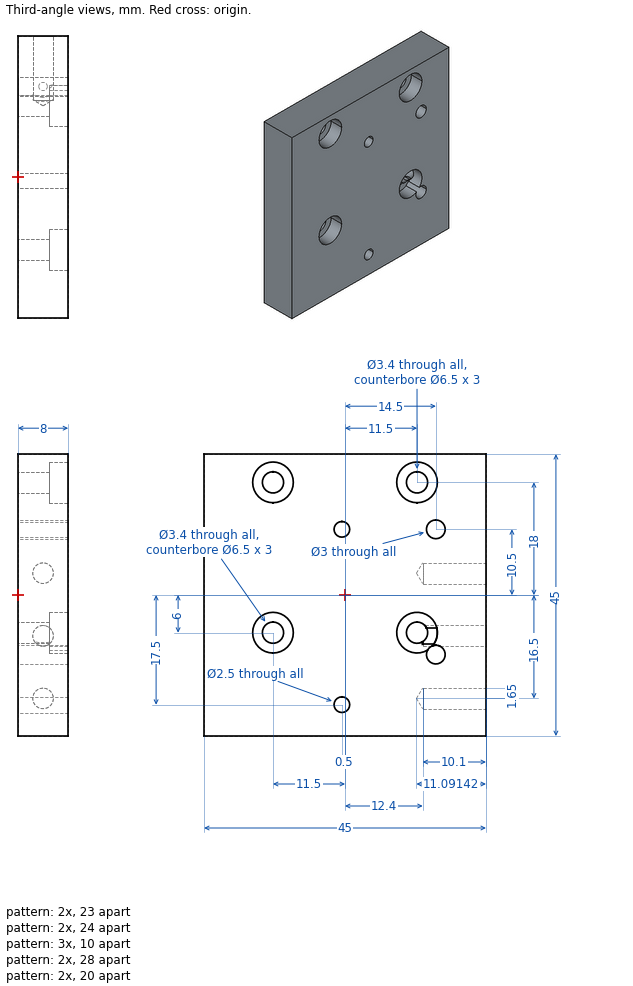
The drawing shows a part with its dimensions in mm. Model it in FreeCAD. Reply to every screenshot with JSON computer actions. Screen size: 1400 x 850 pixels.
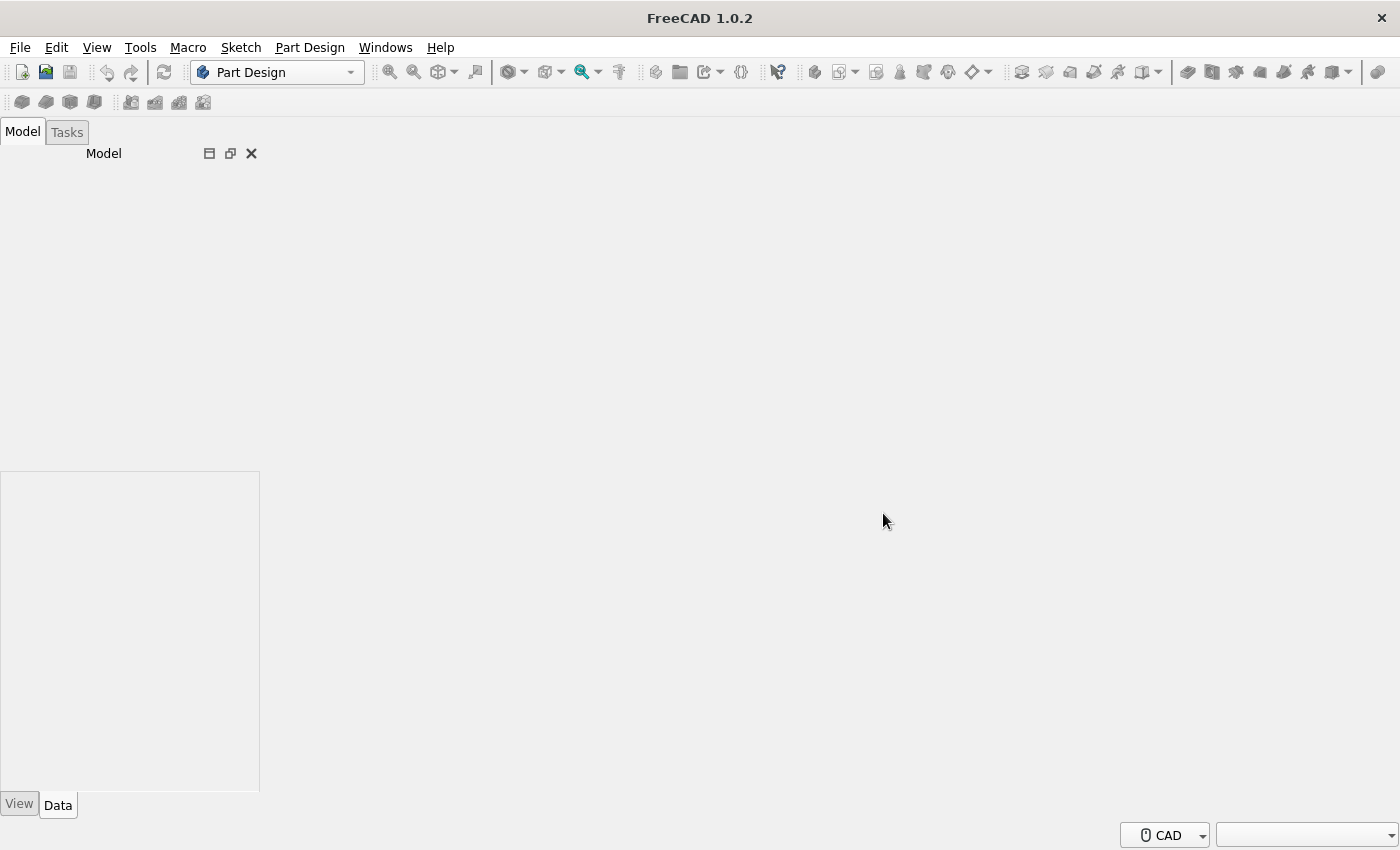
{"action": "key", "text": "ctrl+n"}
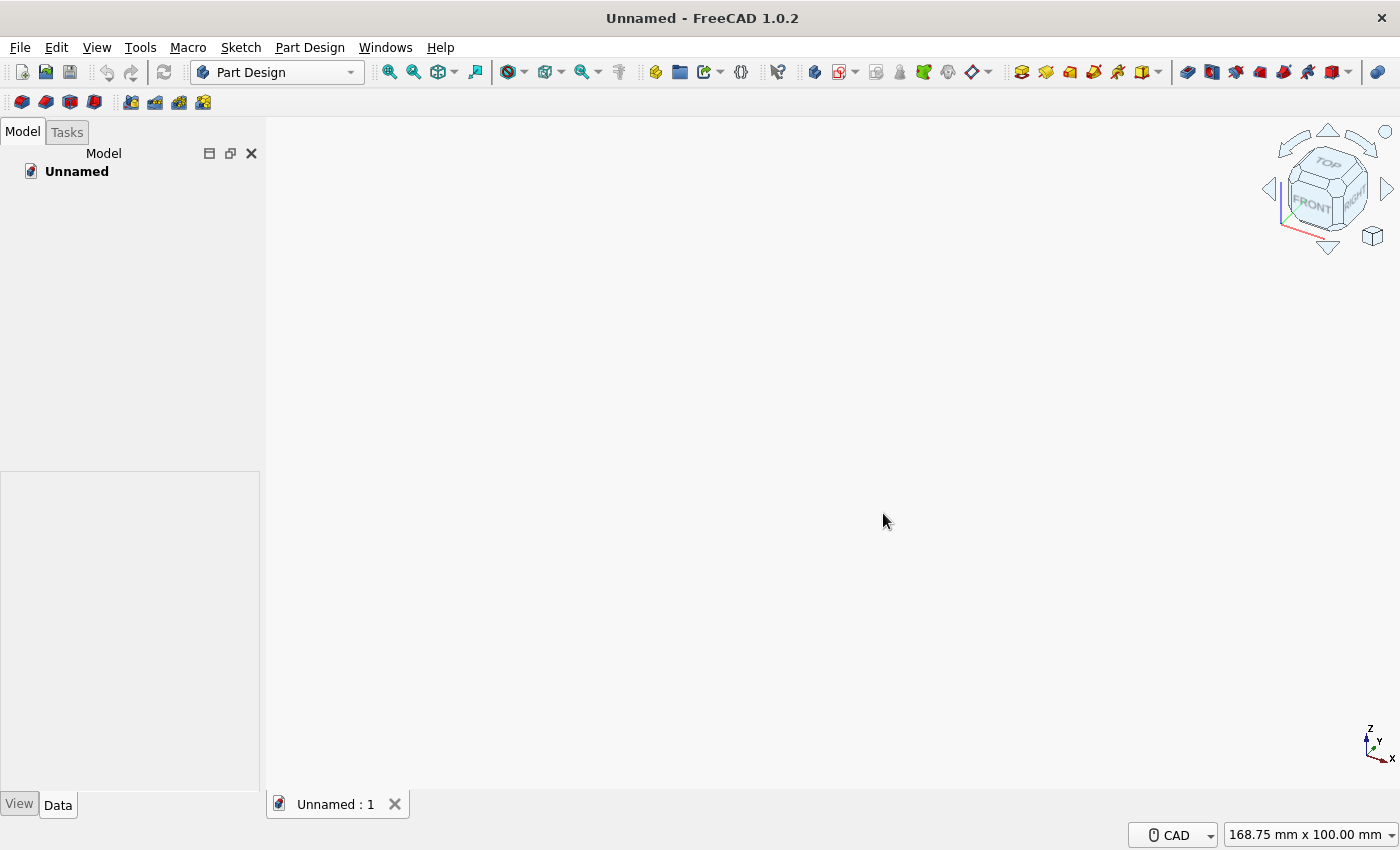
{"action": "left_click", "coordinate": [840, 72]}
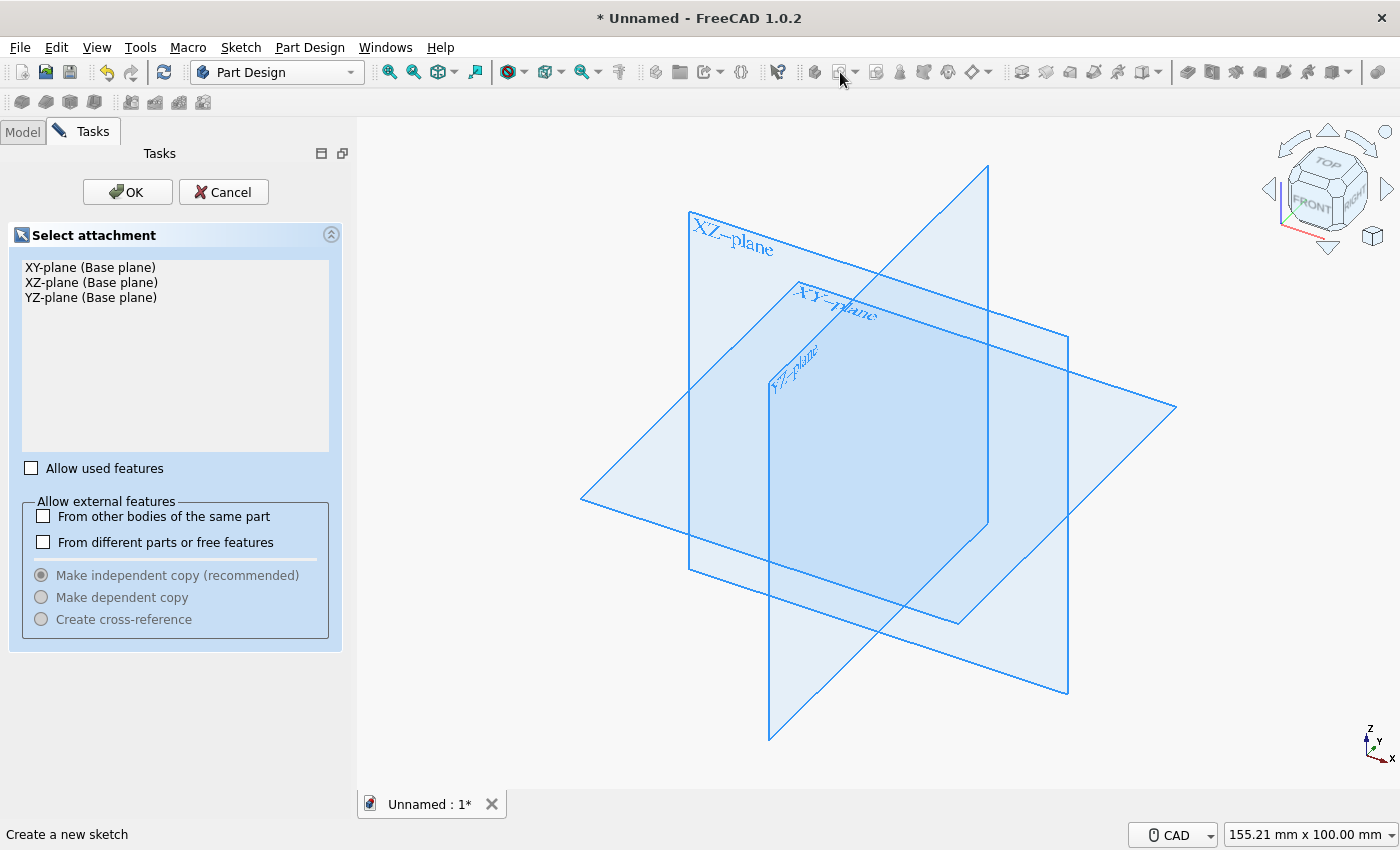
{"action": "left_click", "coordinate": [82, 298]}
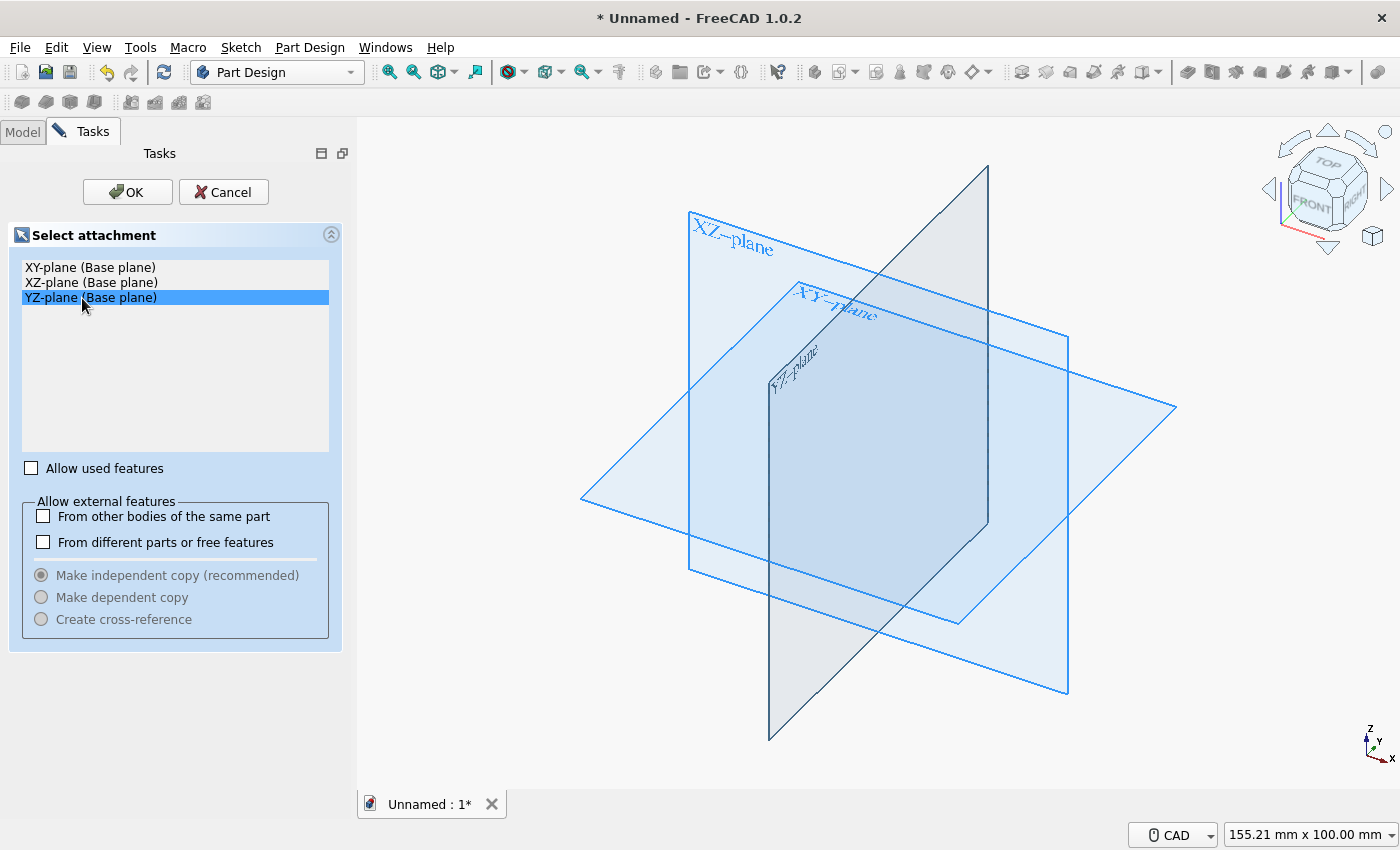
{"action": "left_click", "coordinate": [128, 192]}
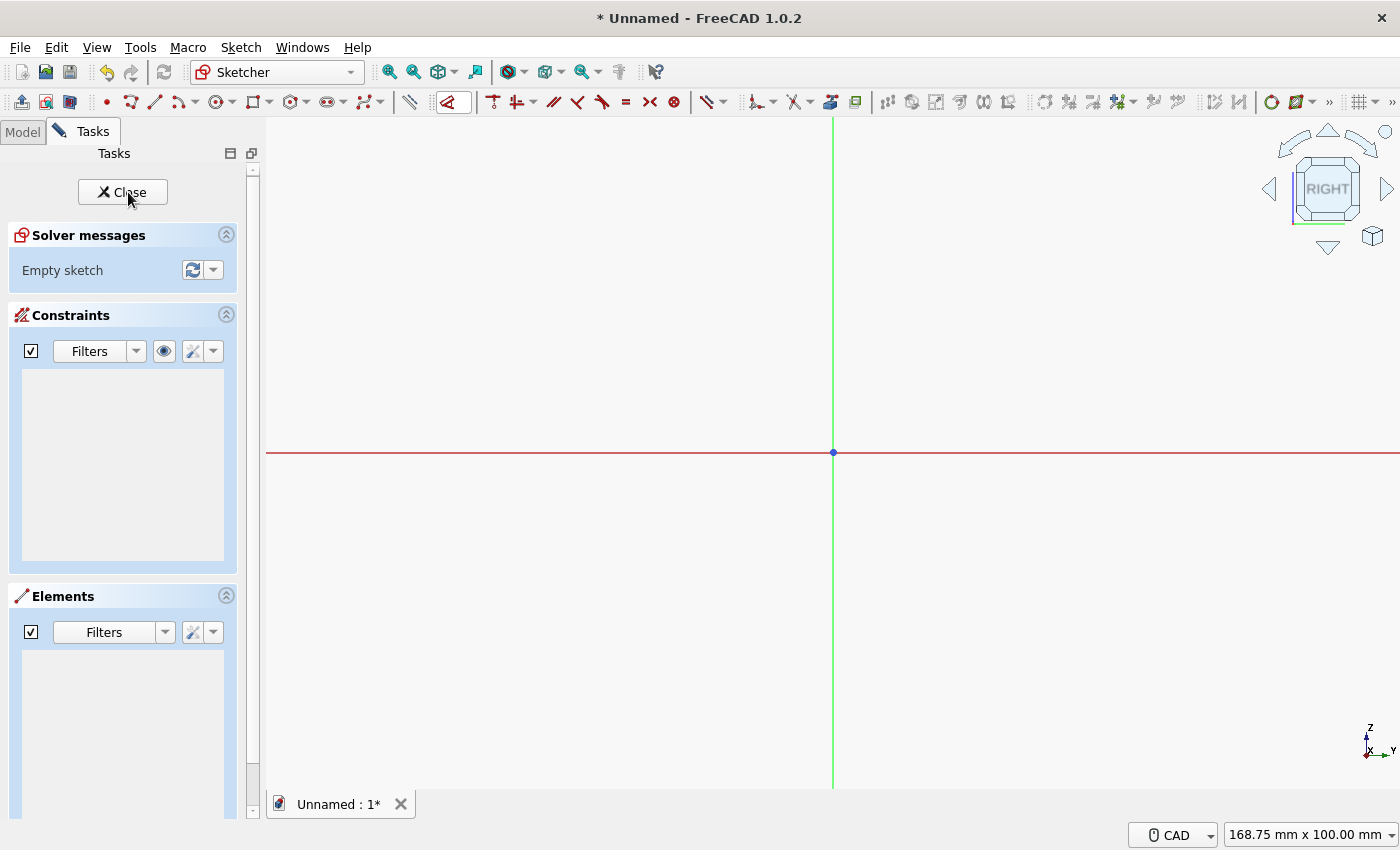
{"action": "scroll", "coordinate": [972, 453], "scroll_direction": "up", "scroll_amount": 2}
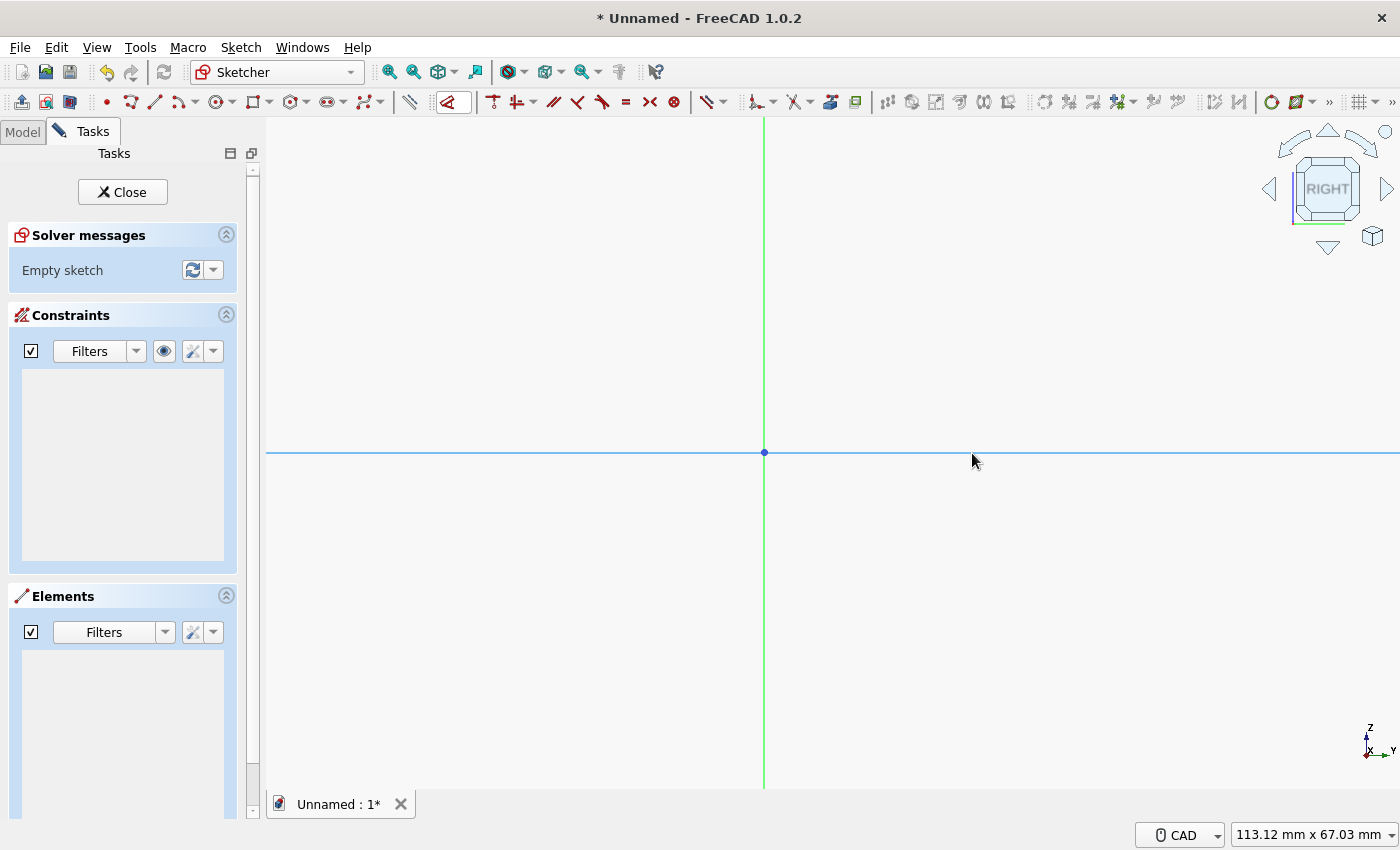
{"action": "key", "text": "g v"}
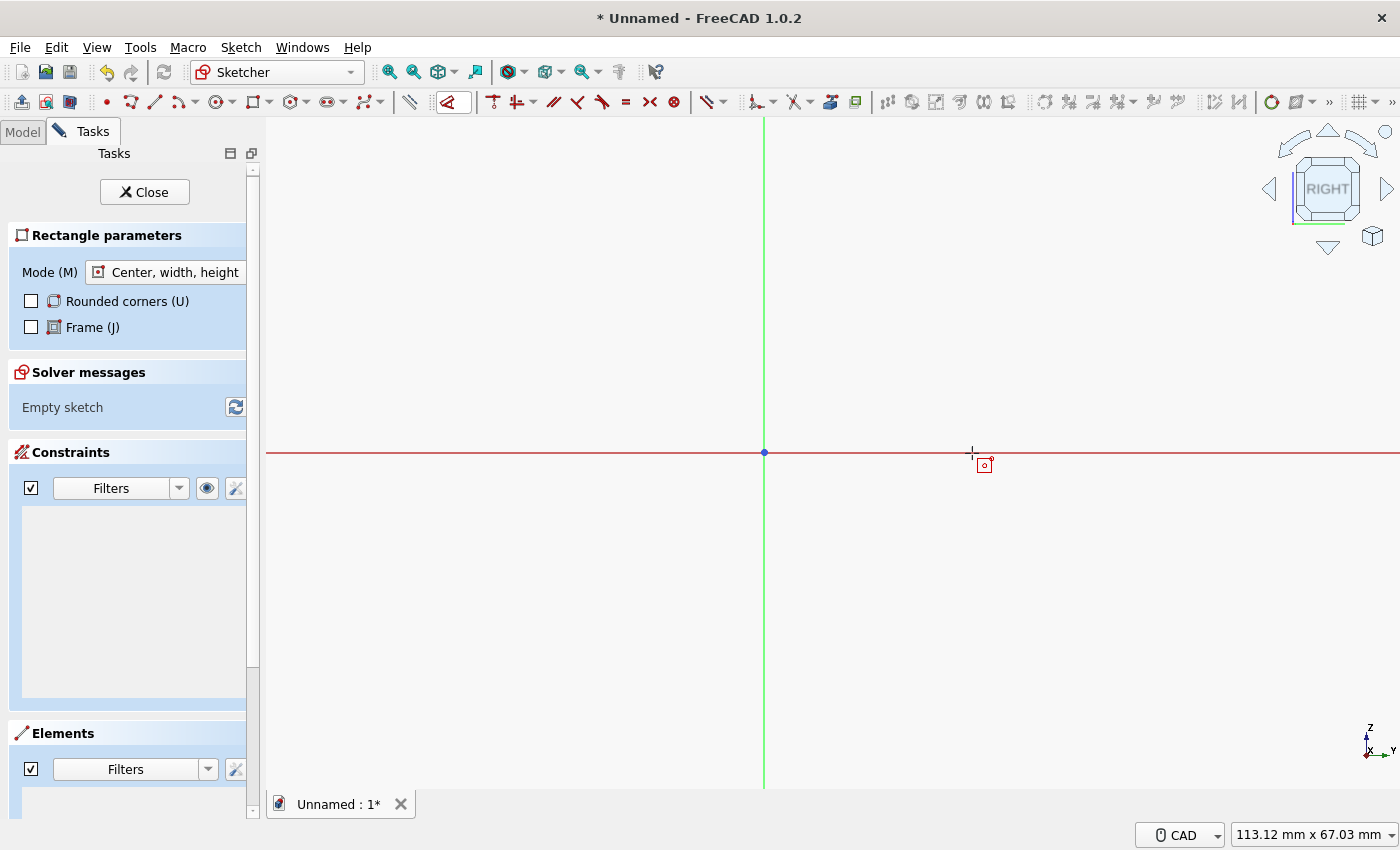
{"action": "left_click", "coordinate": [764, 453]}
{"action": "left_click", "coordinate": [990, 227]}
{"action": "key", "text": "Escape"}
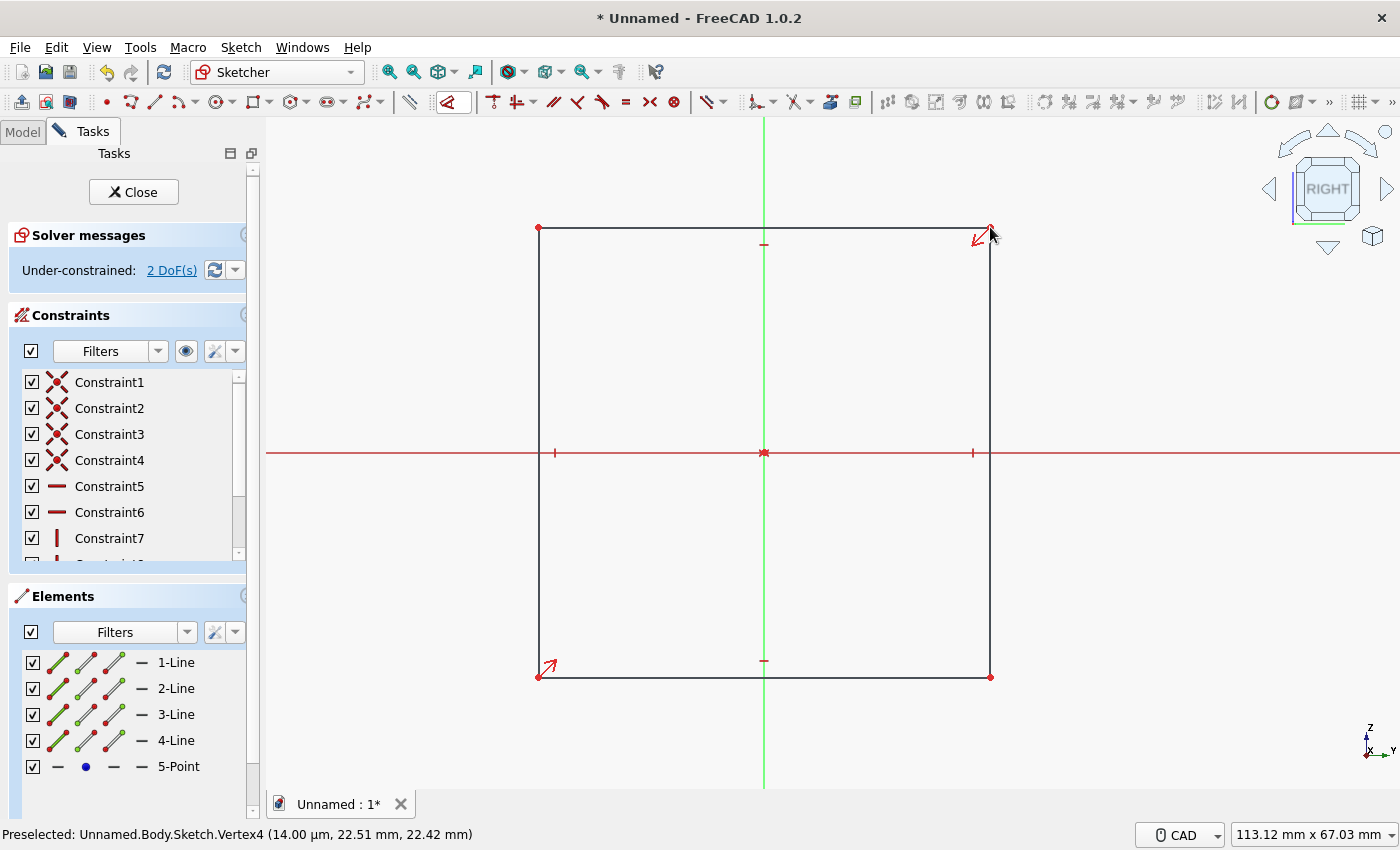
{"action": "key", "text": "d"}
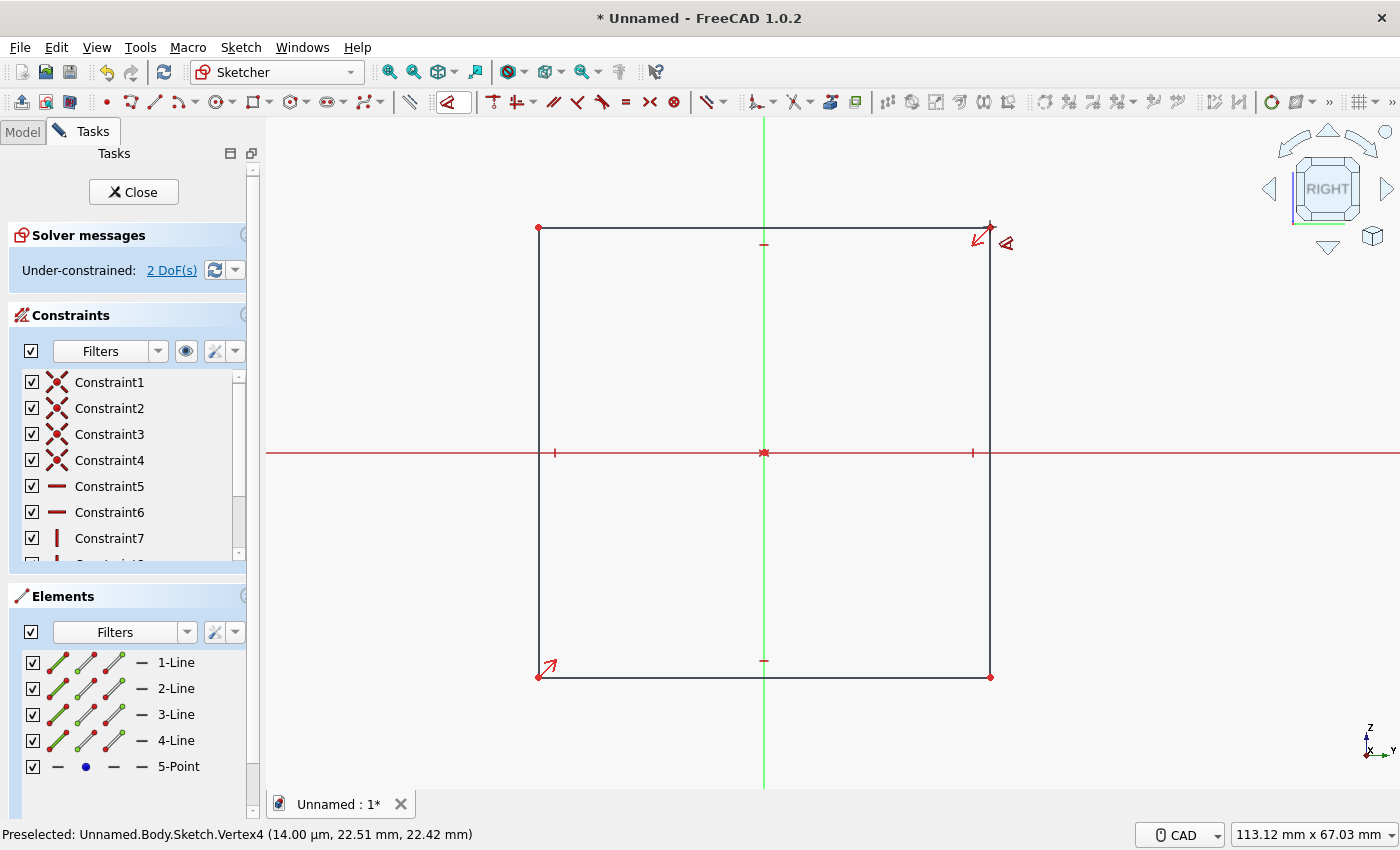
{"action": "left_click", "coordinate": [674, 678]}
{"action": "left_click", "coordinate": [661, 712]}